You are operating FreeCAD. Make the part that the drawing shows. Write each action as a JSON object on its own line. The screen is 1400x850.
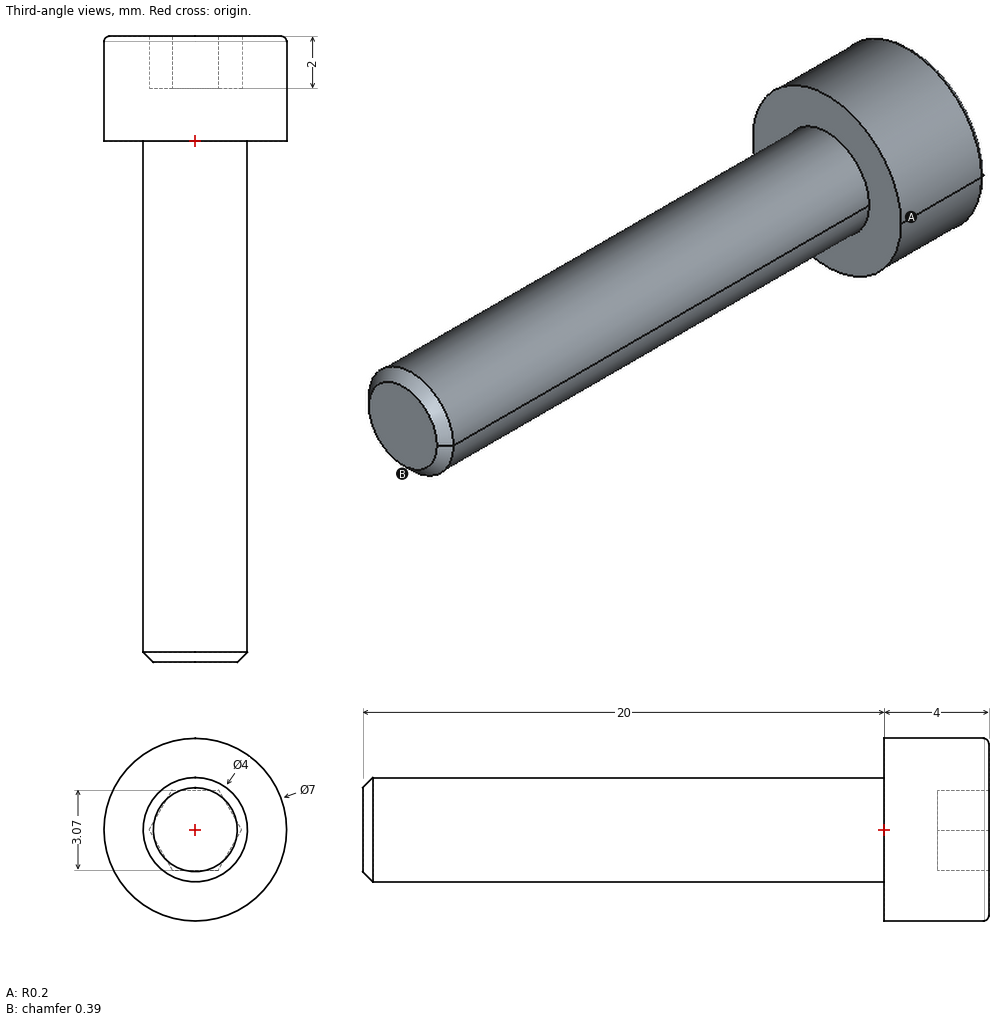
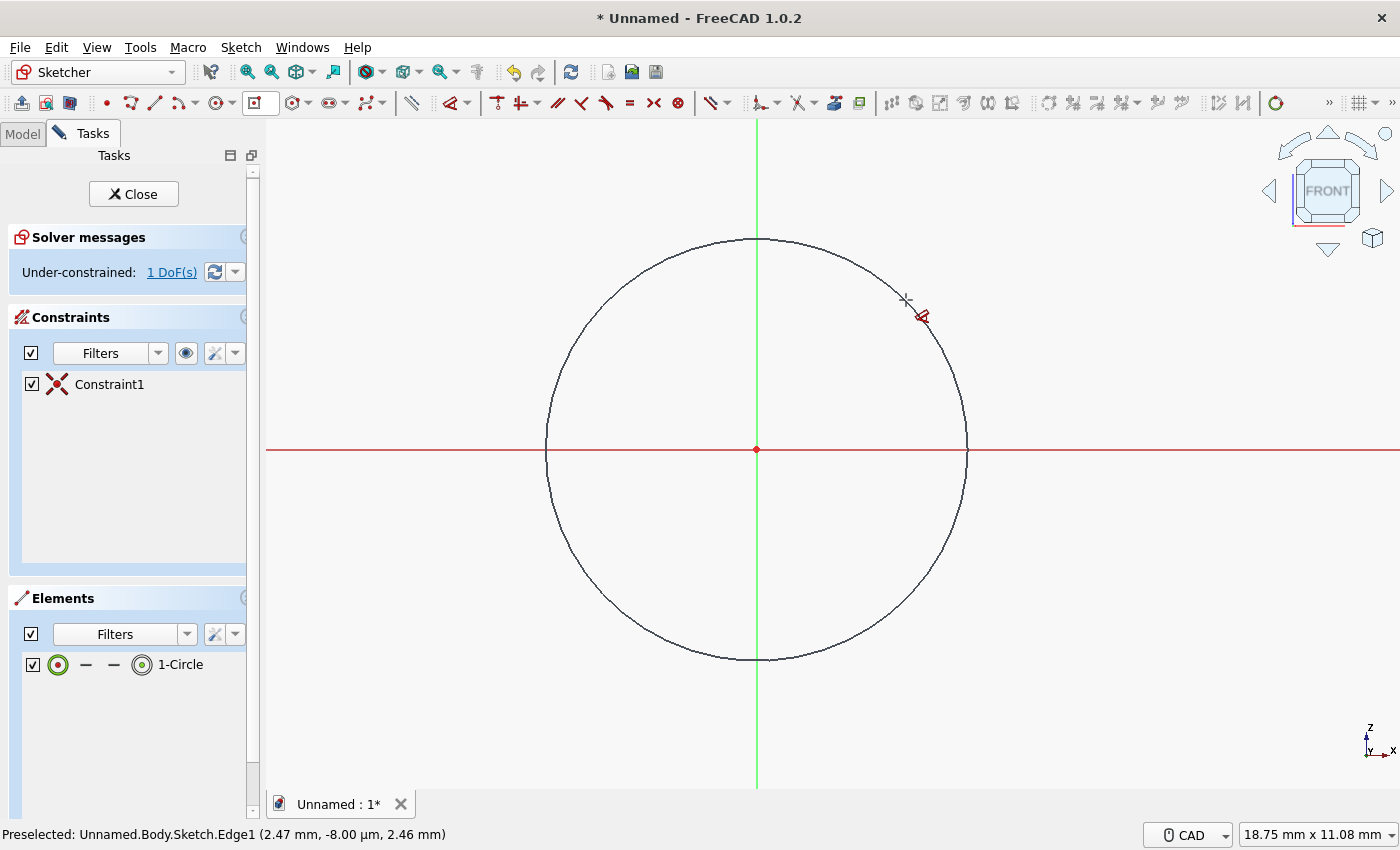
{"action": "left_click", "coordinate": [905, 300]}
{"action": "left_click", "coordinate": [927, 277]}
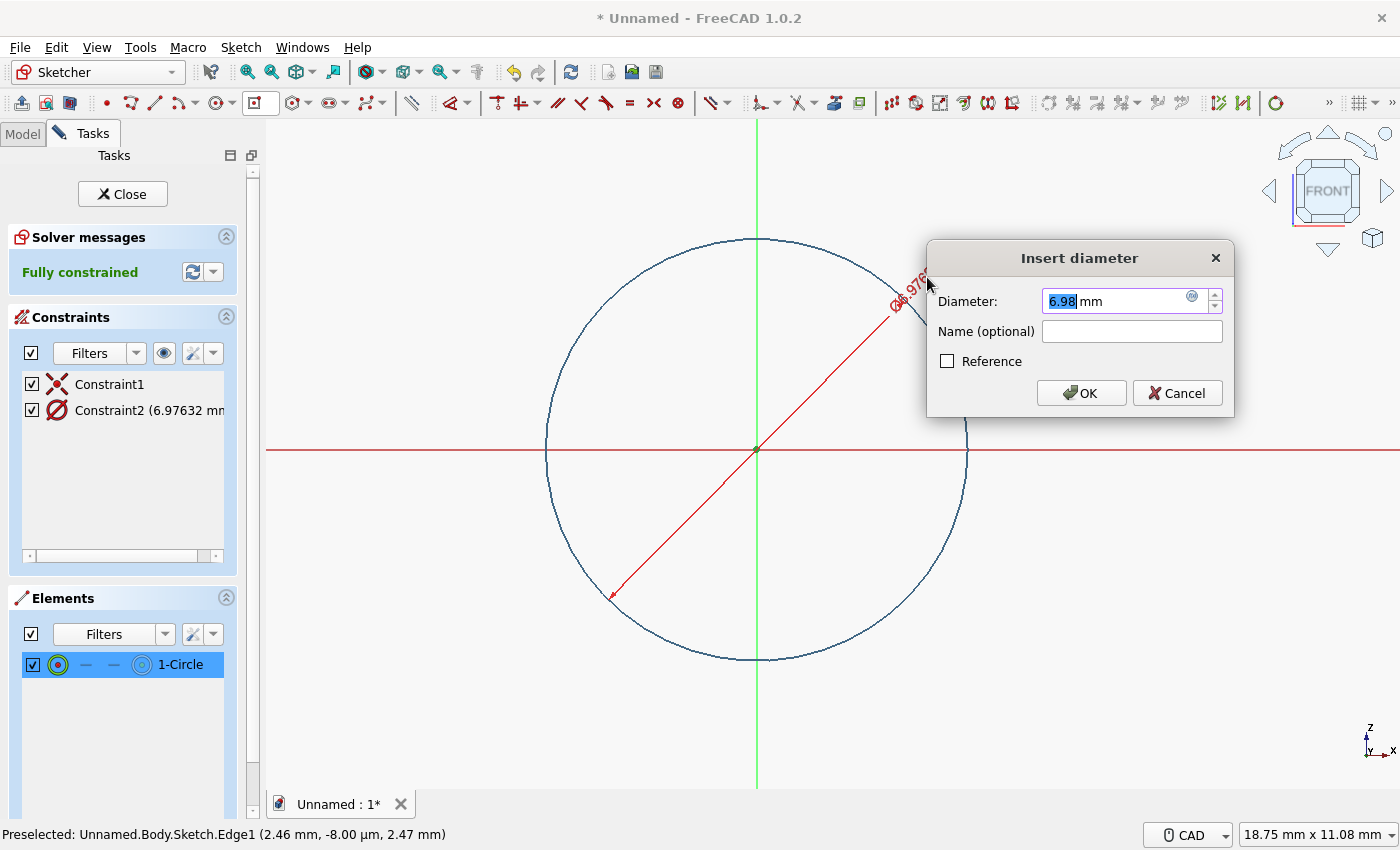
{"action": "type", "text": "7"}
{"action": "key", "text": "Return"}
{"action": "key", "text": "Escape"}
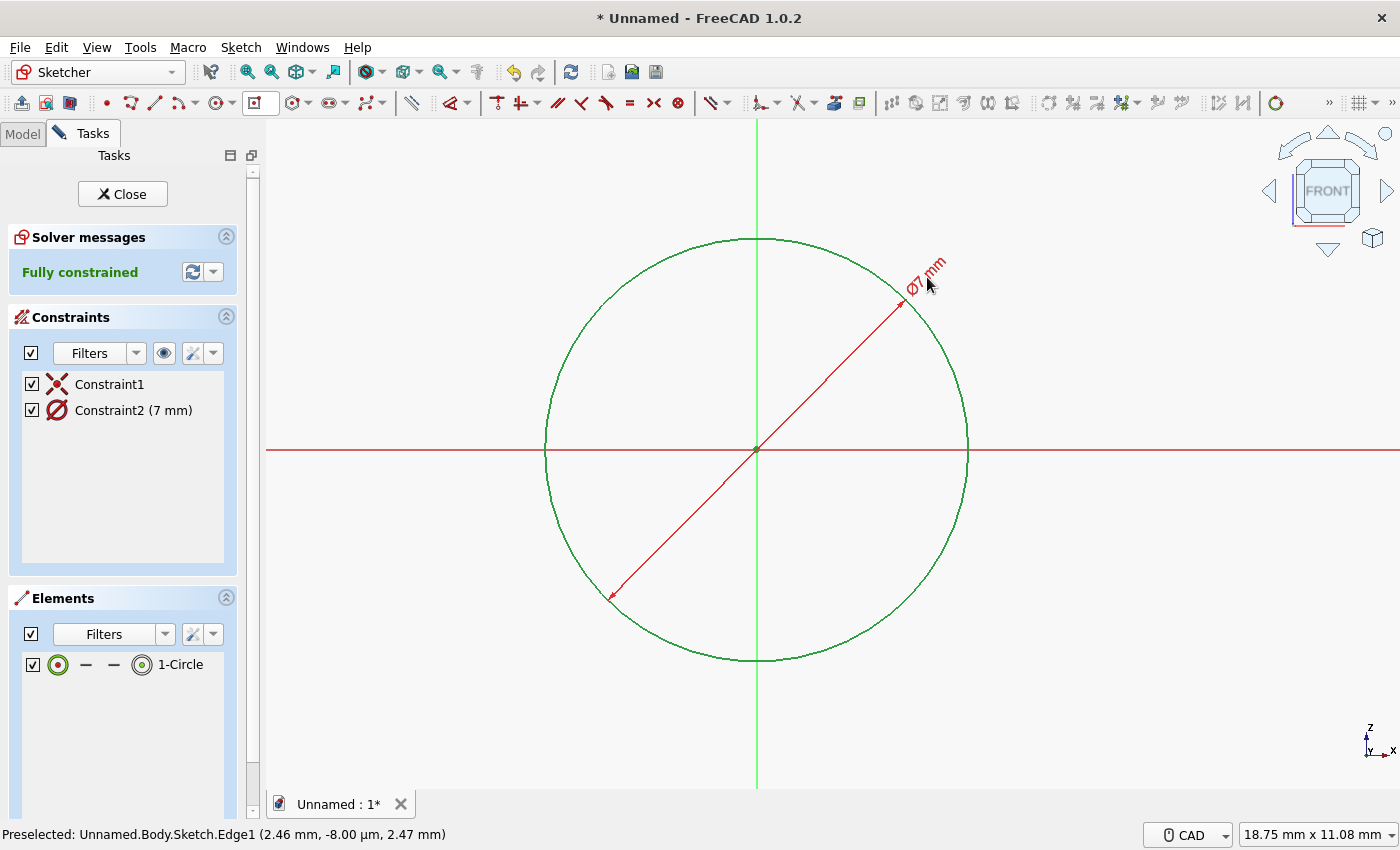
{"action": "left_click", "coordinate": [123, 194]}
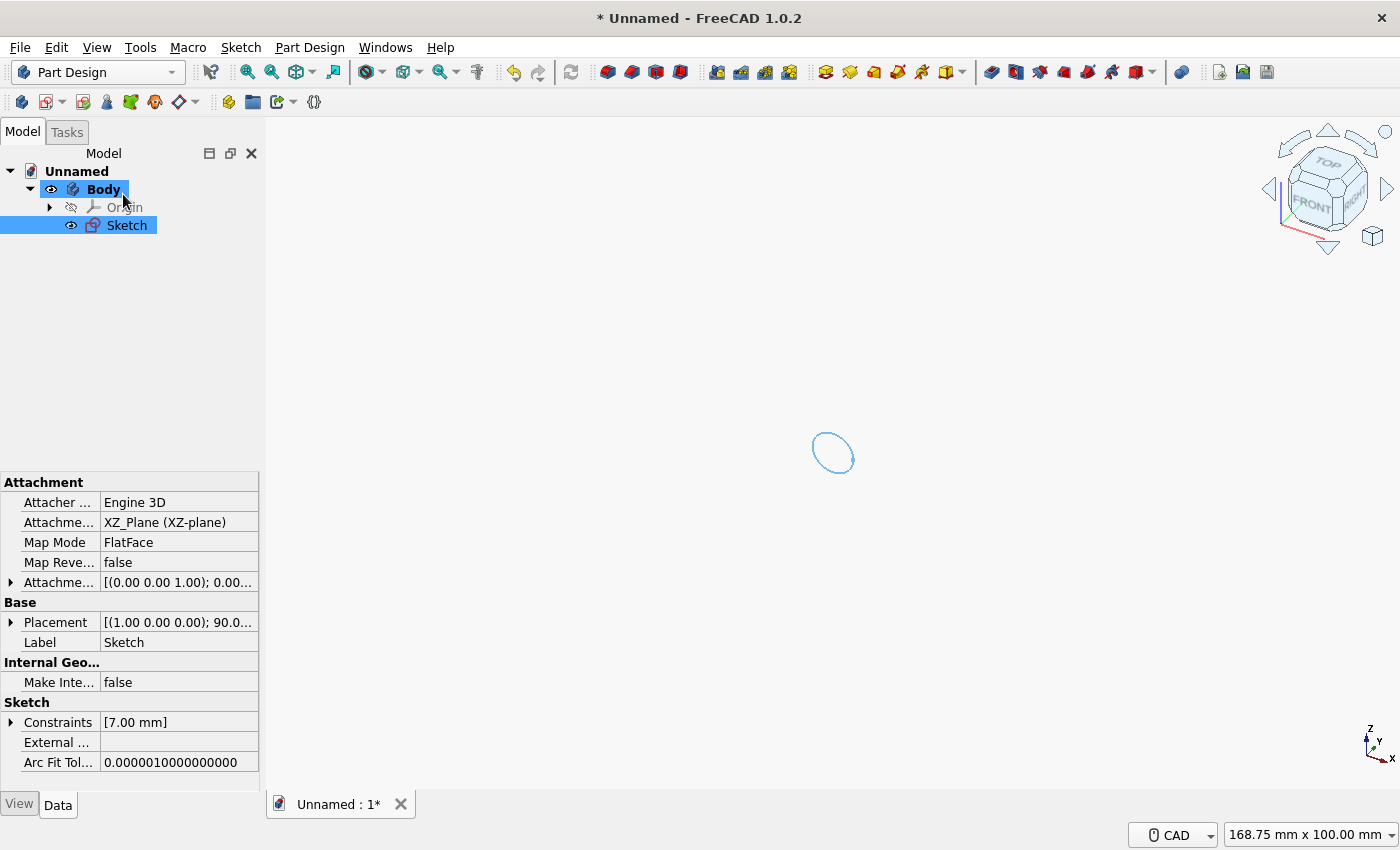
{"action": "left_click", "coordinate": [826, 72]}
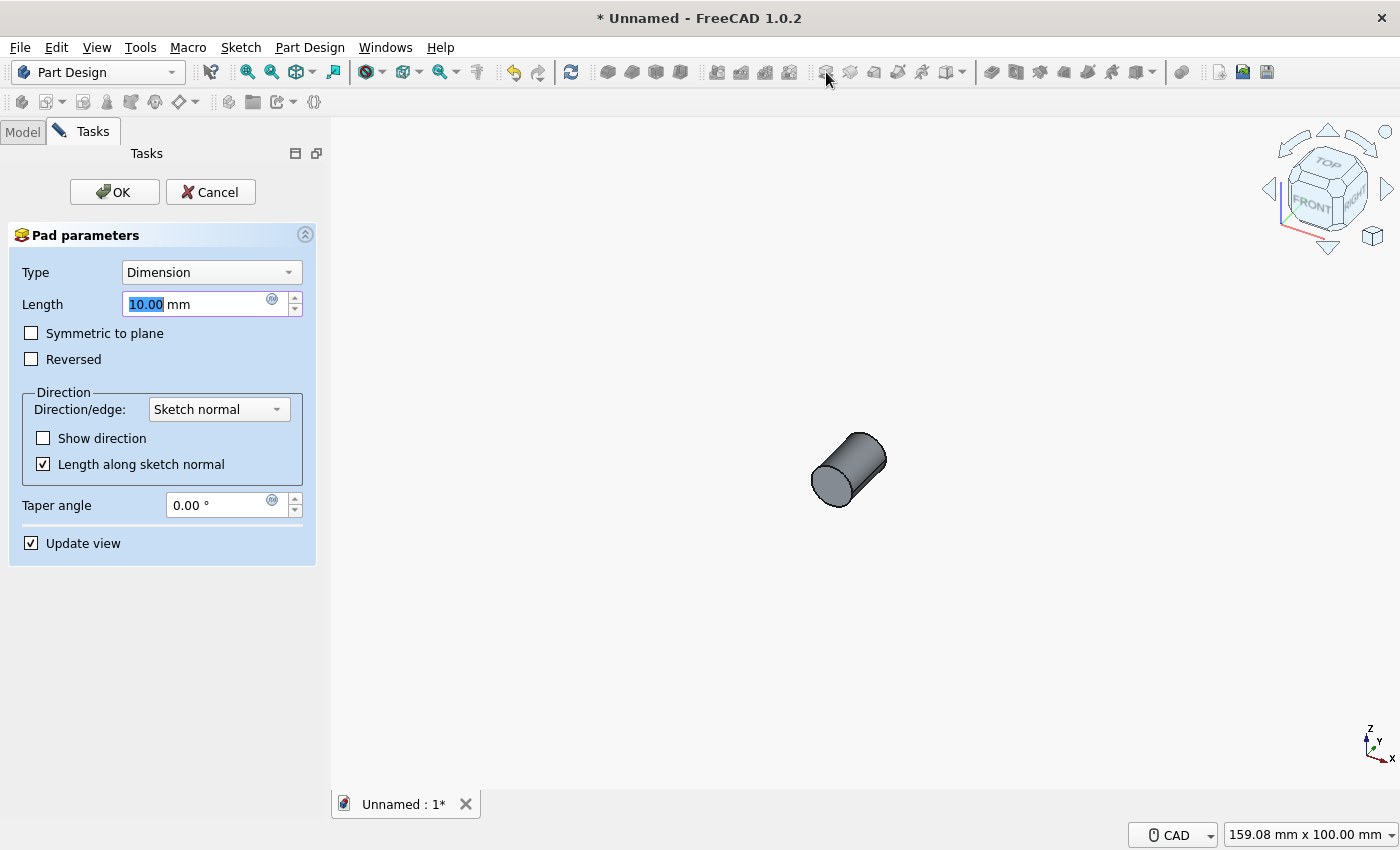
{"action": "type", "text": "4"}
{"action": "key", "text": "Tab"}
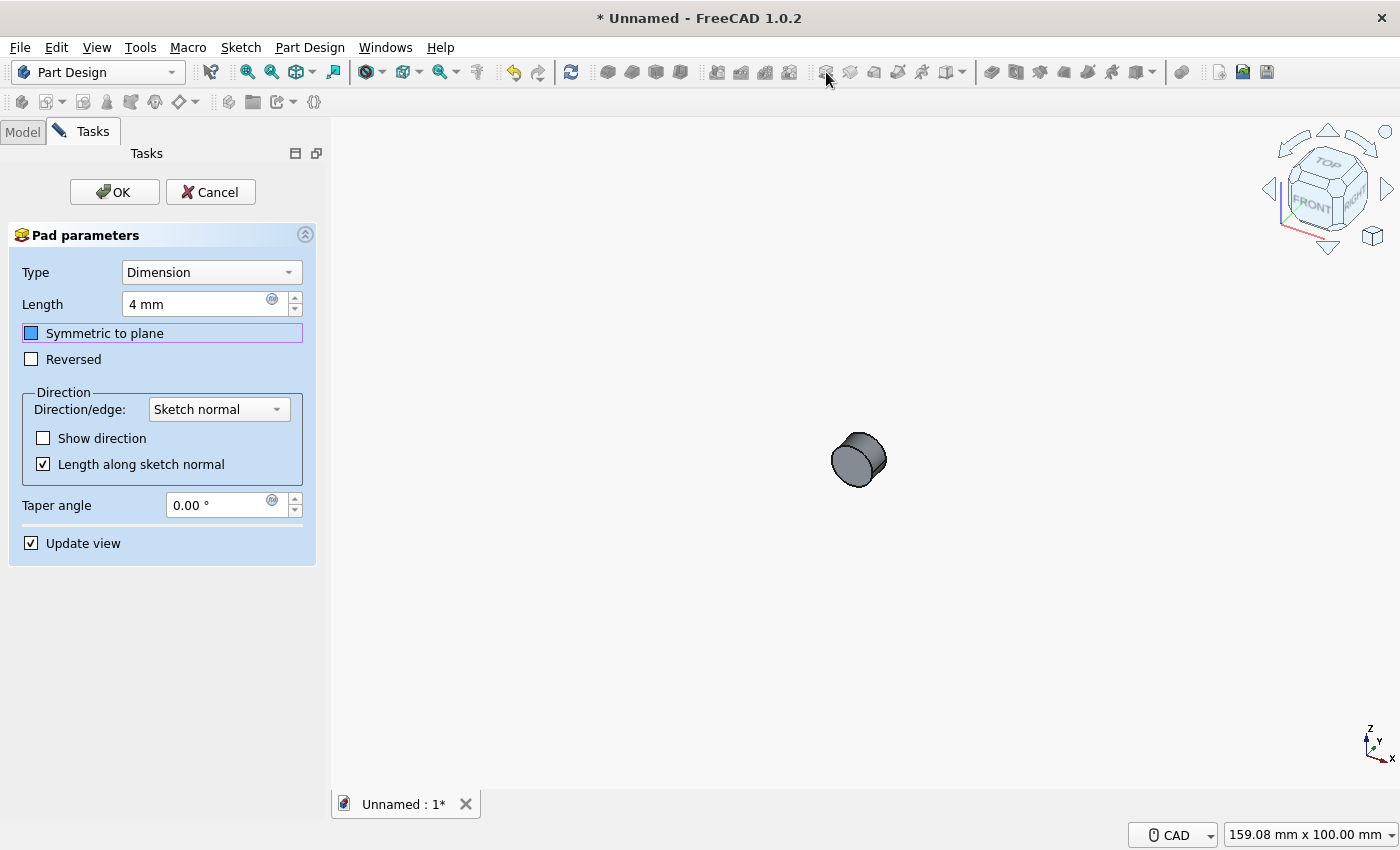
{"action": "left_click", "coordinate": [30, 359]}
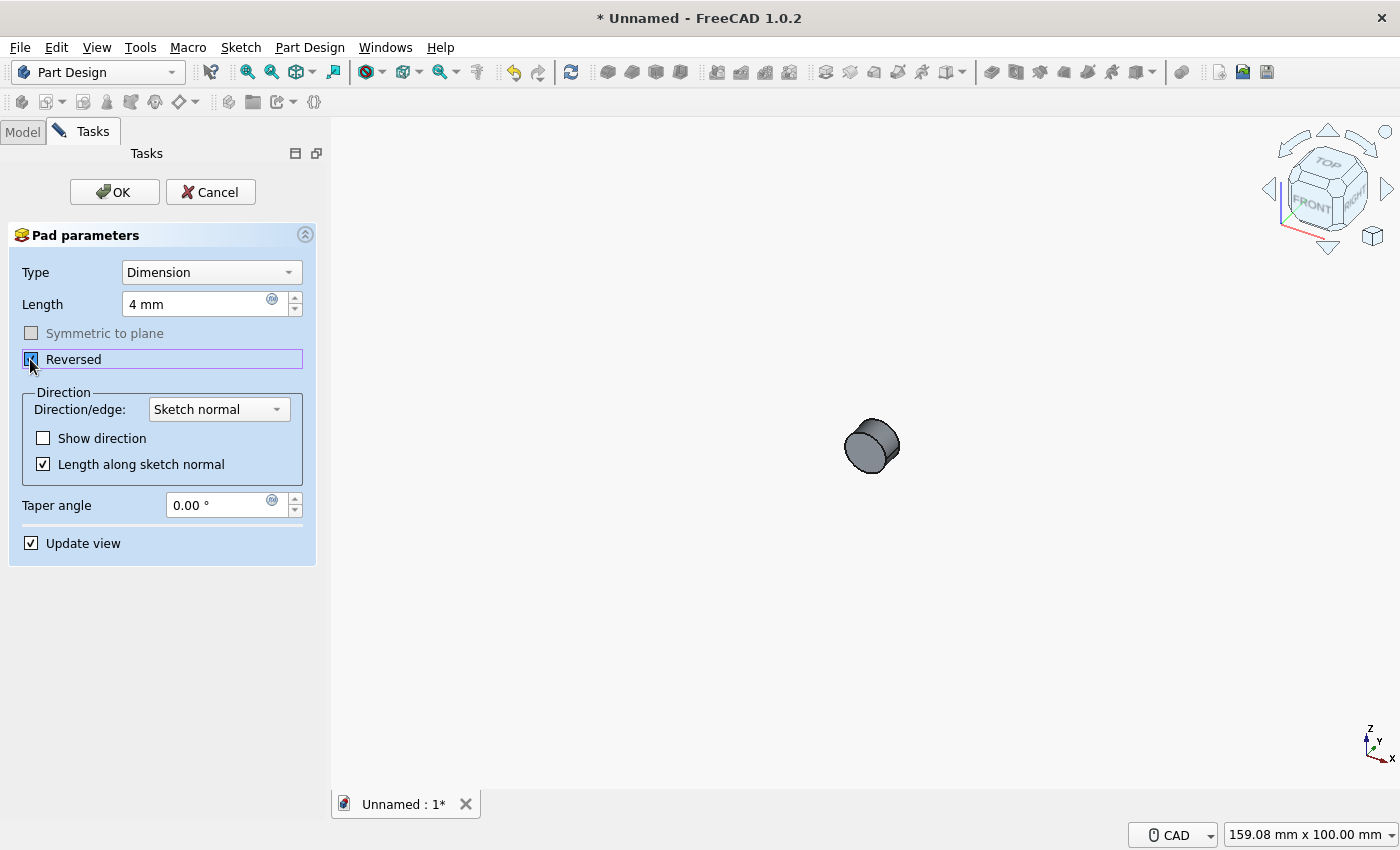
{"action": "left_click", "coordinate": [115, 192]}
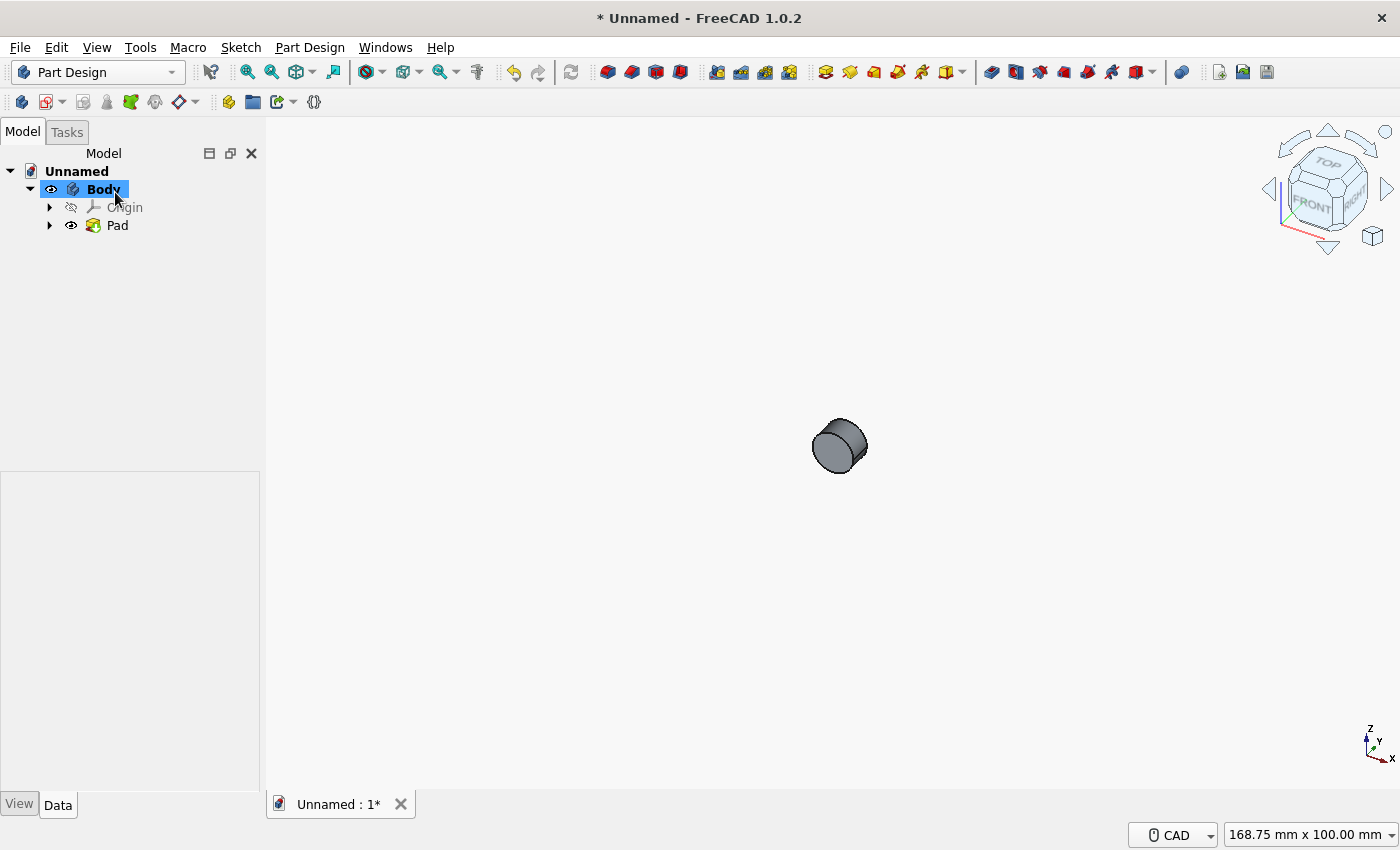
{"action": "key", "text": "v f"}